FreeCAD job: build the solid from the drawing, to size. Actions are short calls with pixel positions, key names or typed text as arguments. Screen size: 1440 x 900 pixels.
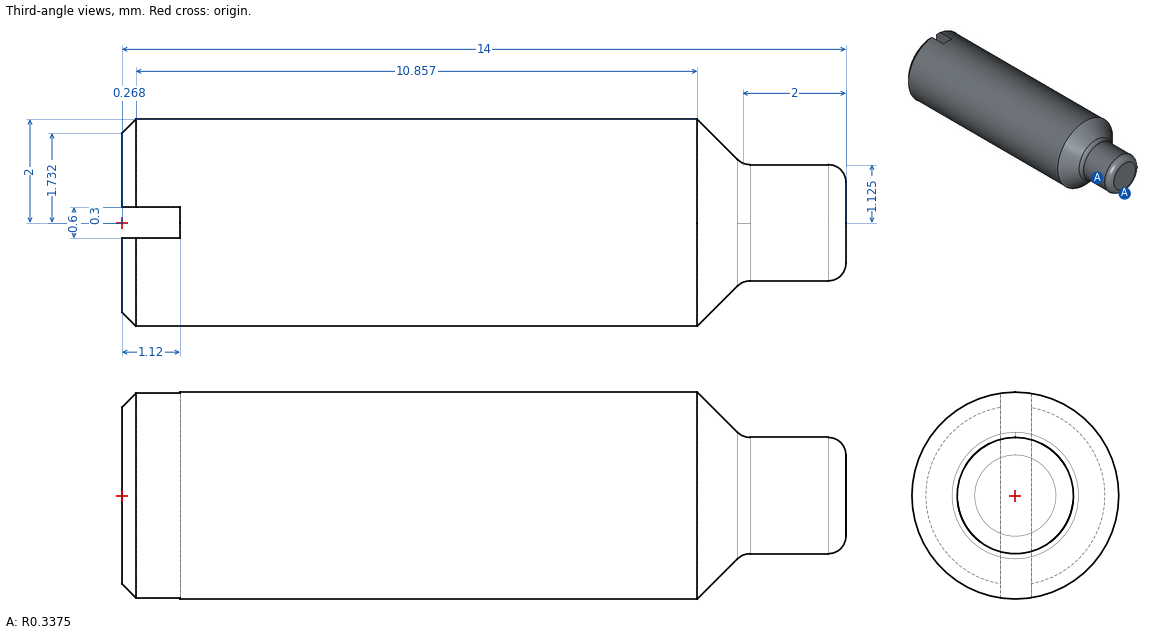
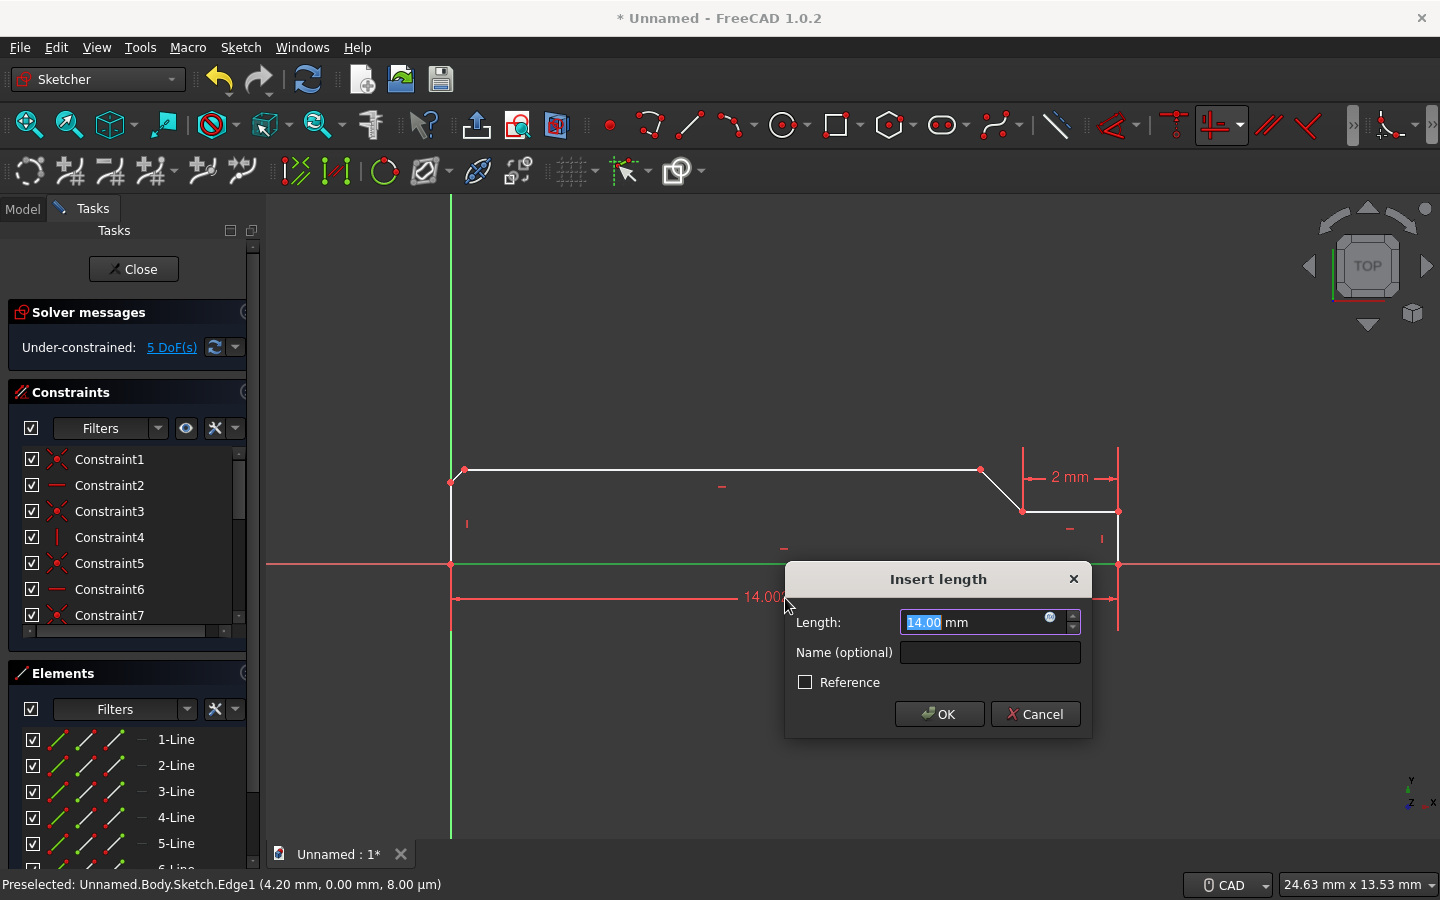
text(14)
key(Return)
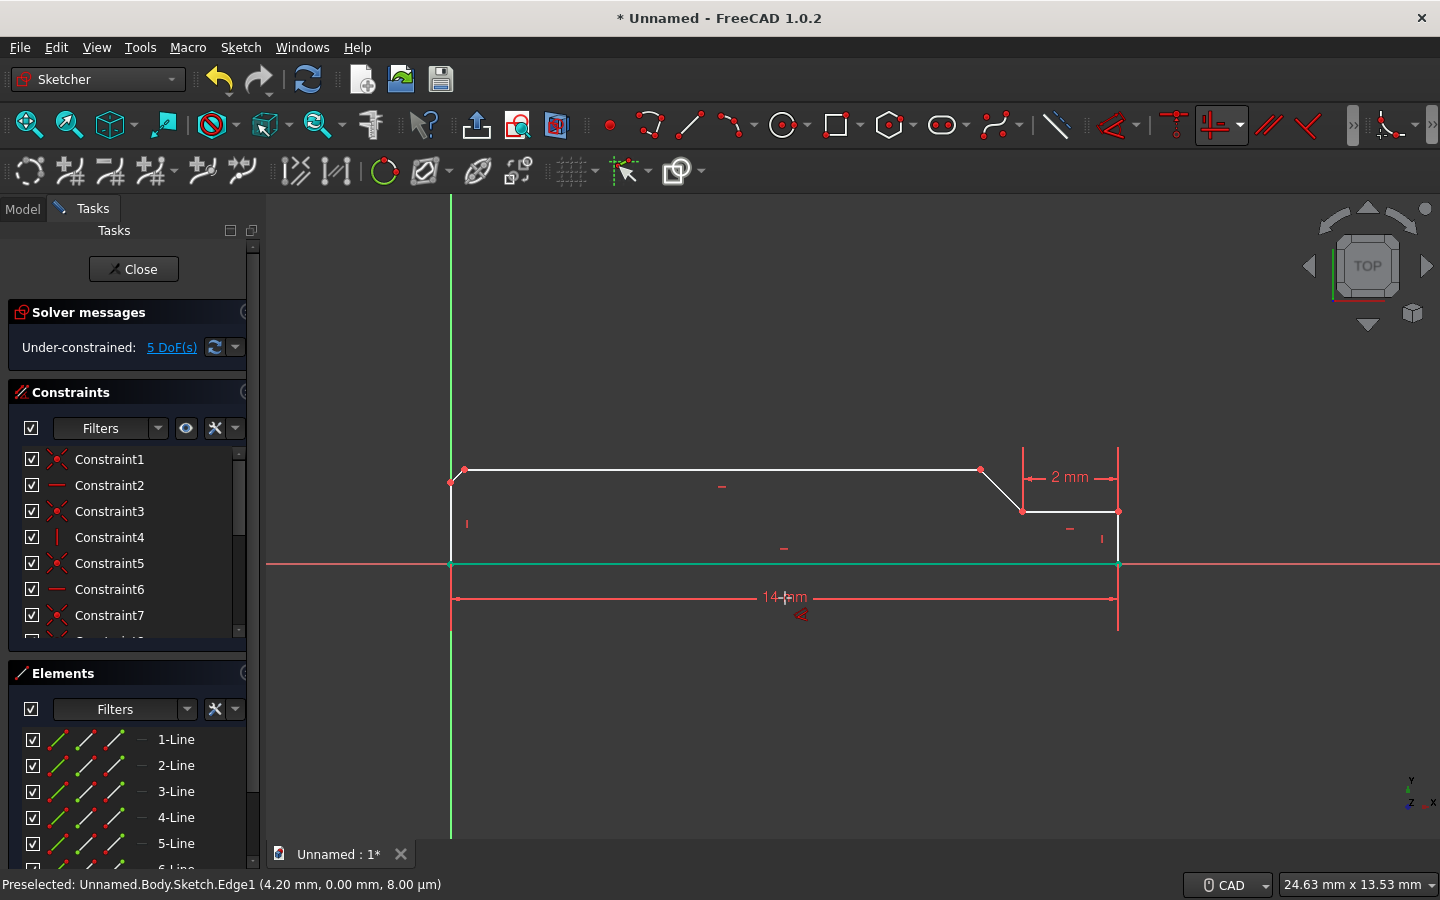
click(981, 470)
click(417, 517)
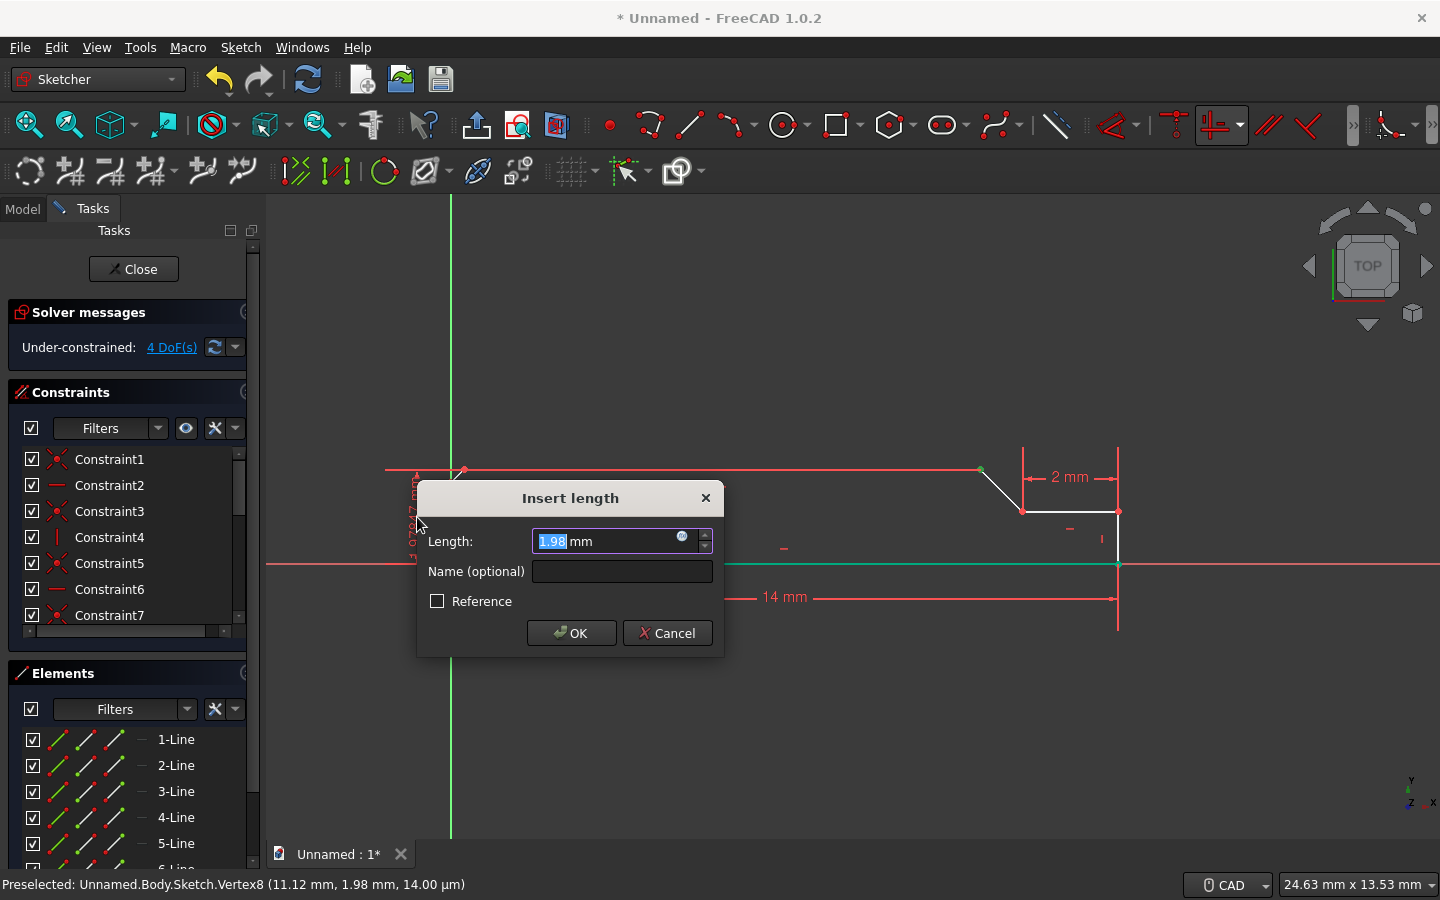
text(2)
key(Return)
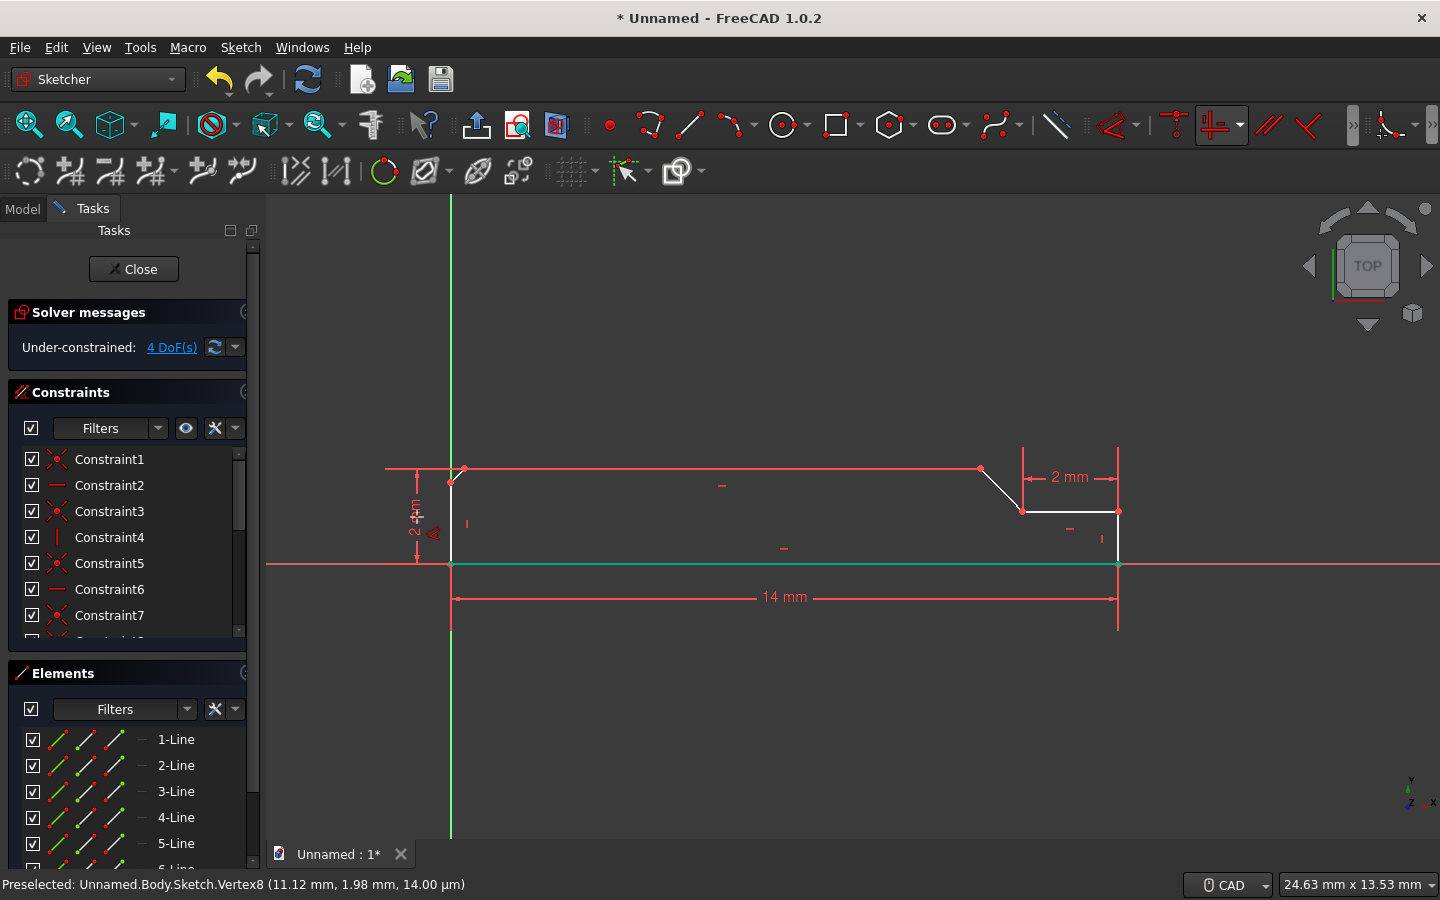
click(1118, 549)
click(1152, 538)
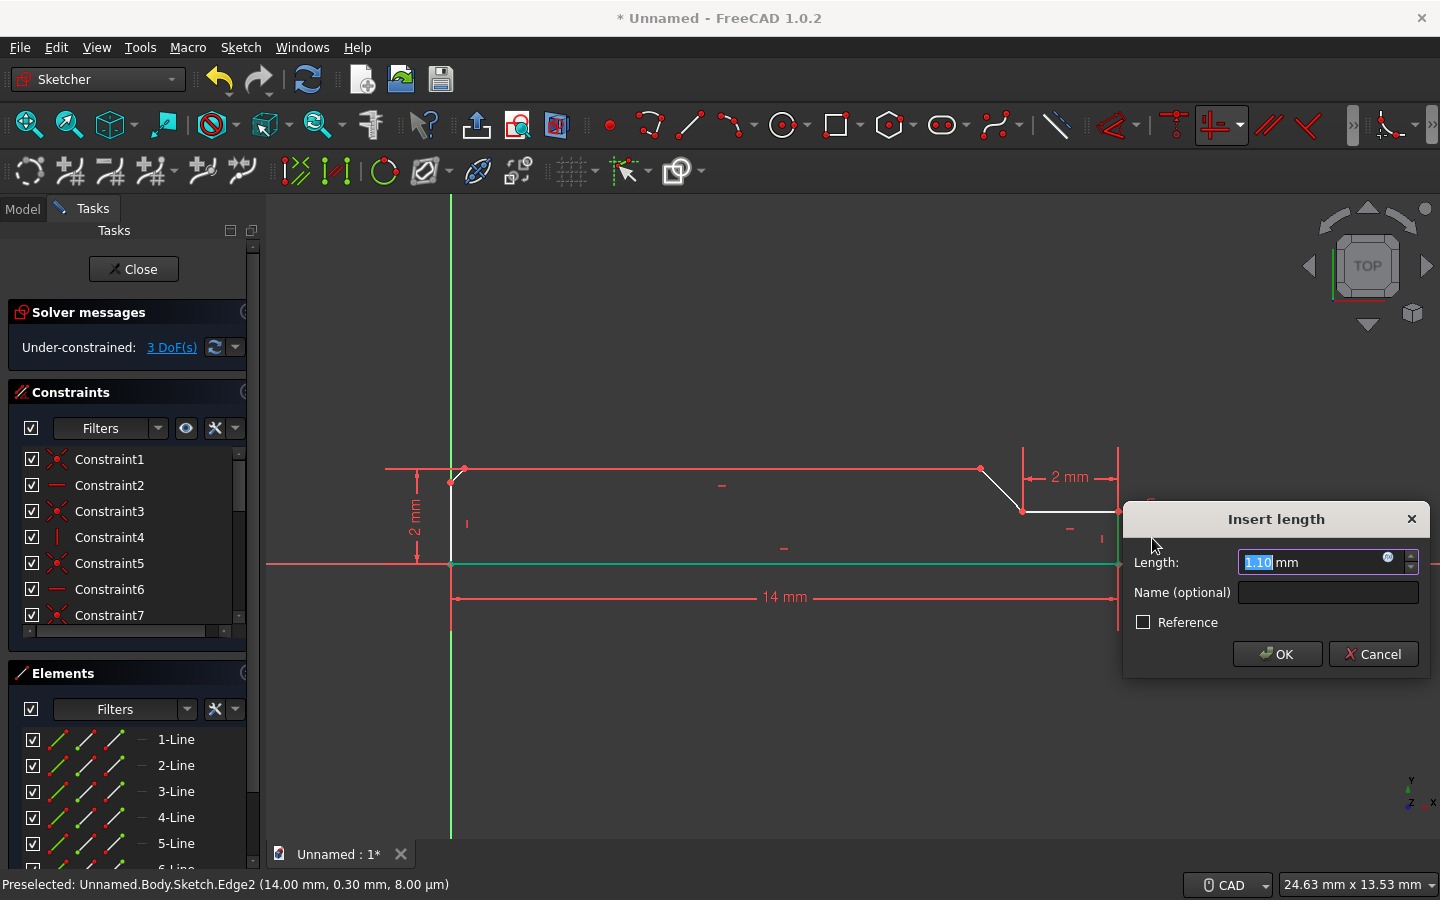
text(1.125)
key(Return)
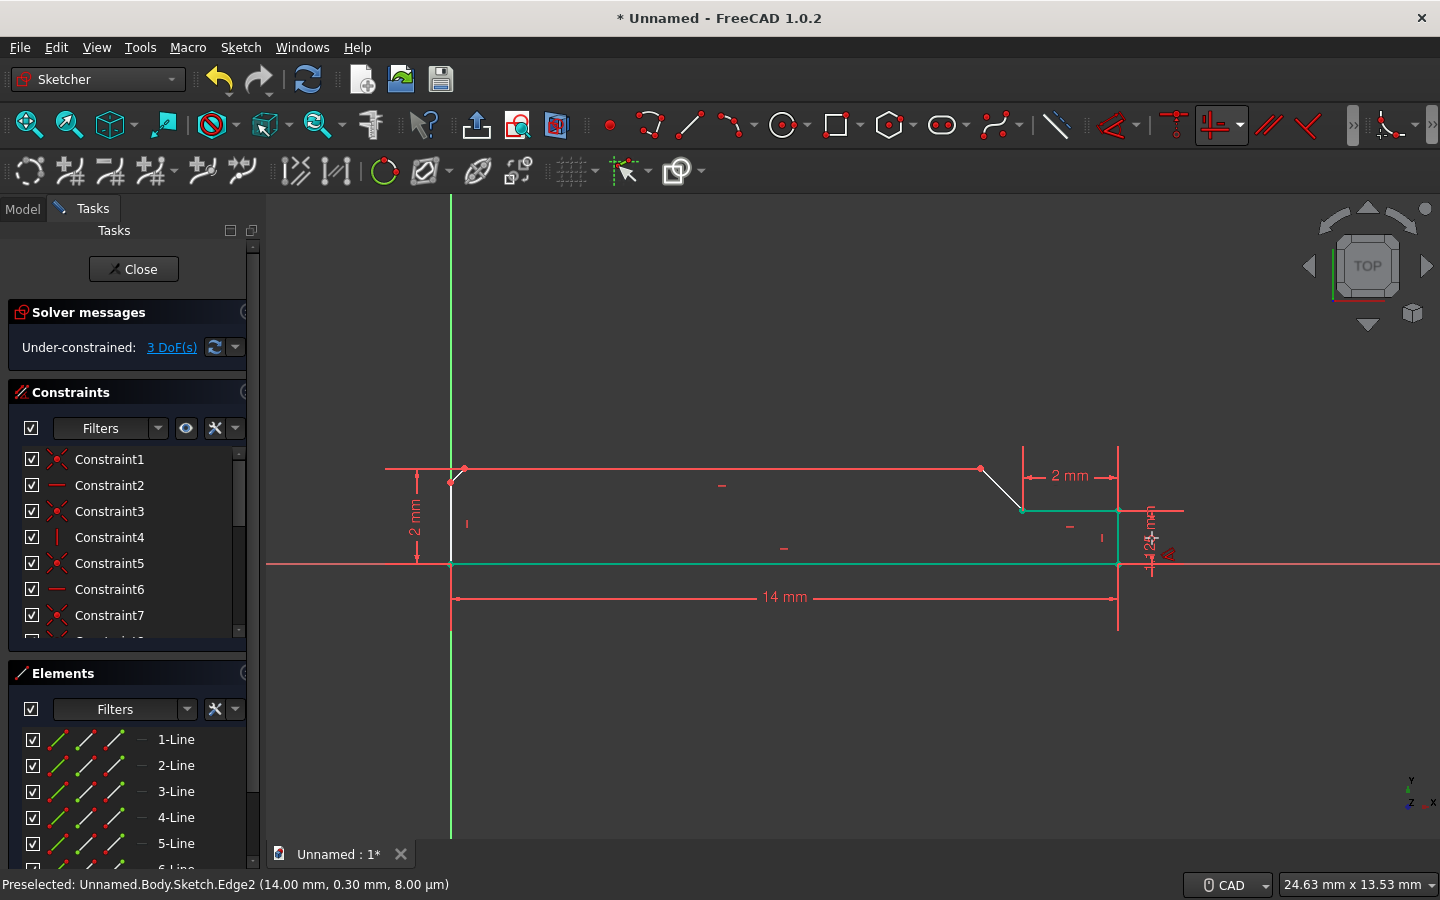
click(451, 507)
click(417, 542)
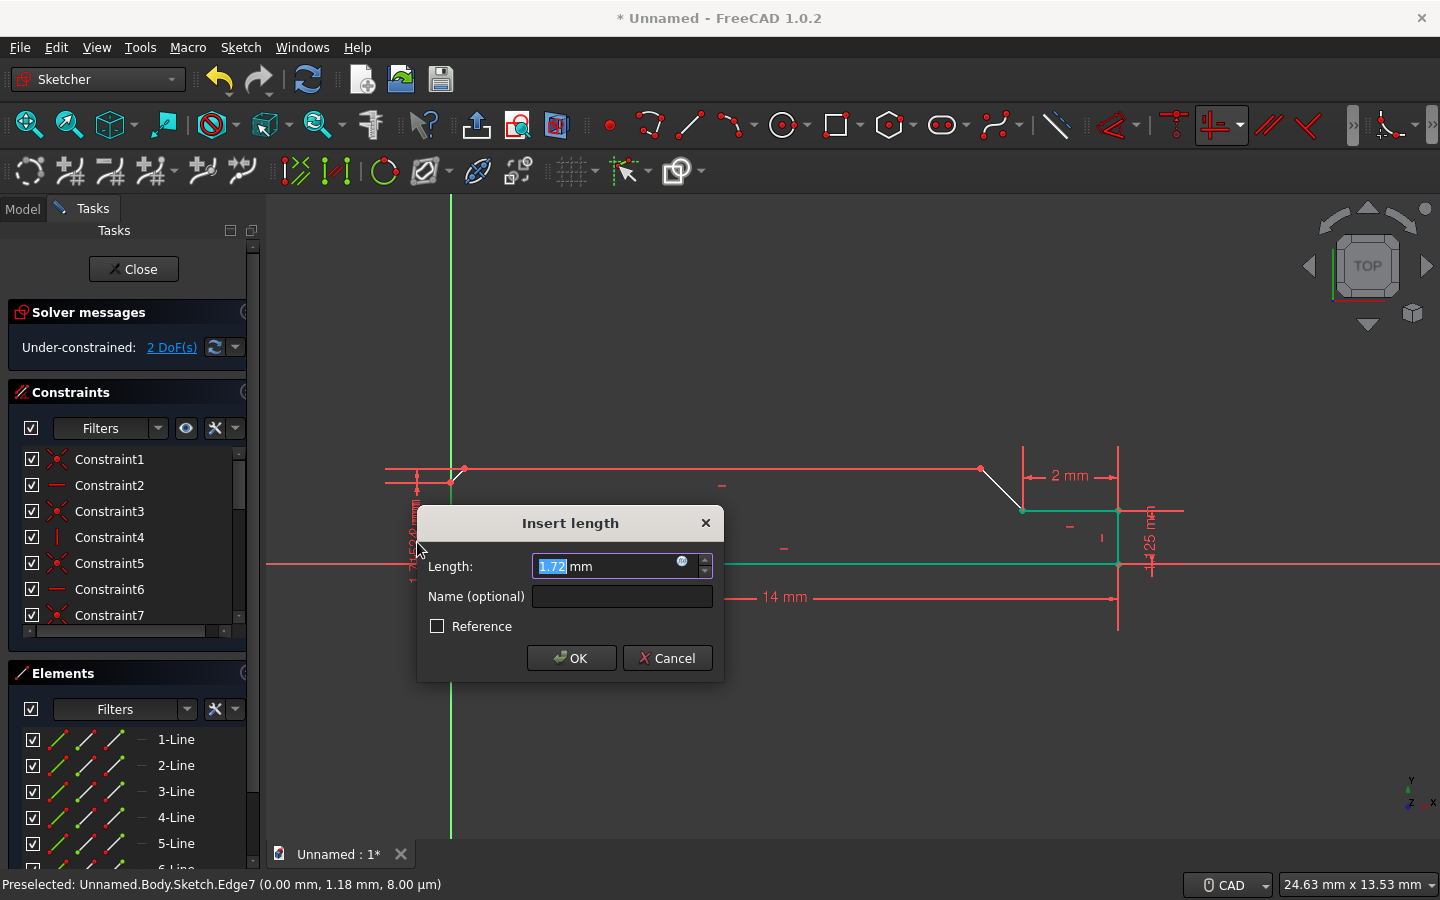
text(1.732)
key(Return)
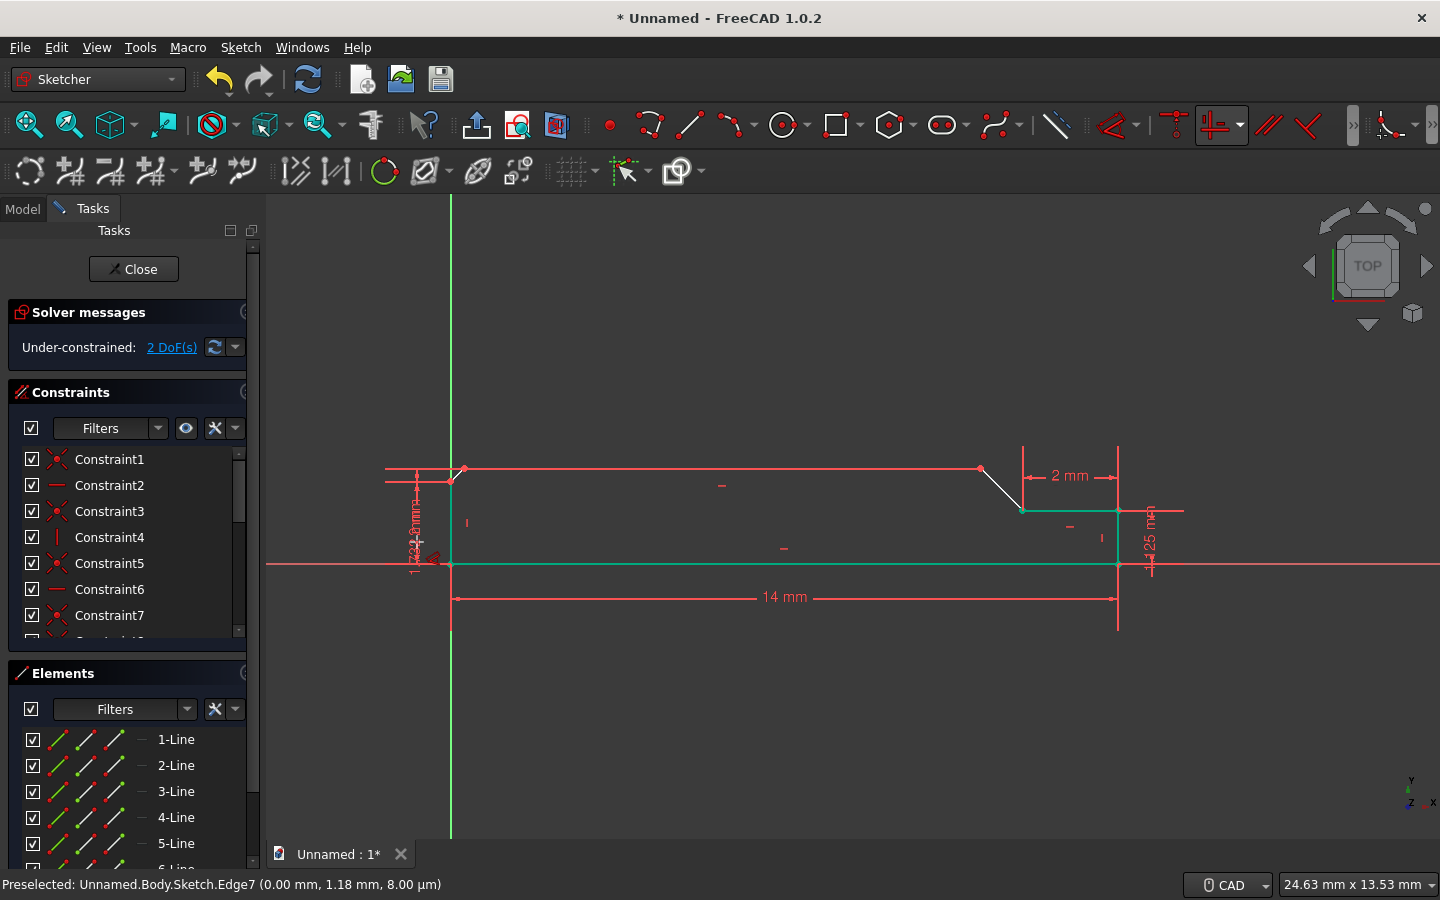
click(826, 469)
click(722, 435)